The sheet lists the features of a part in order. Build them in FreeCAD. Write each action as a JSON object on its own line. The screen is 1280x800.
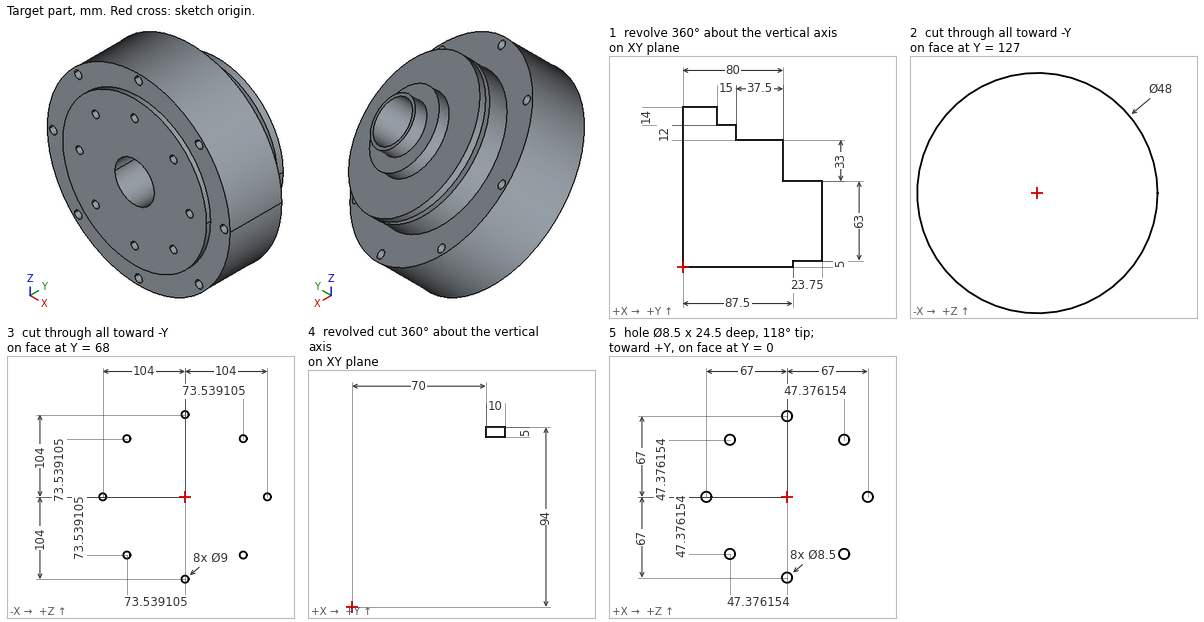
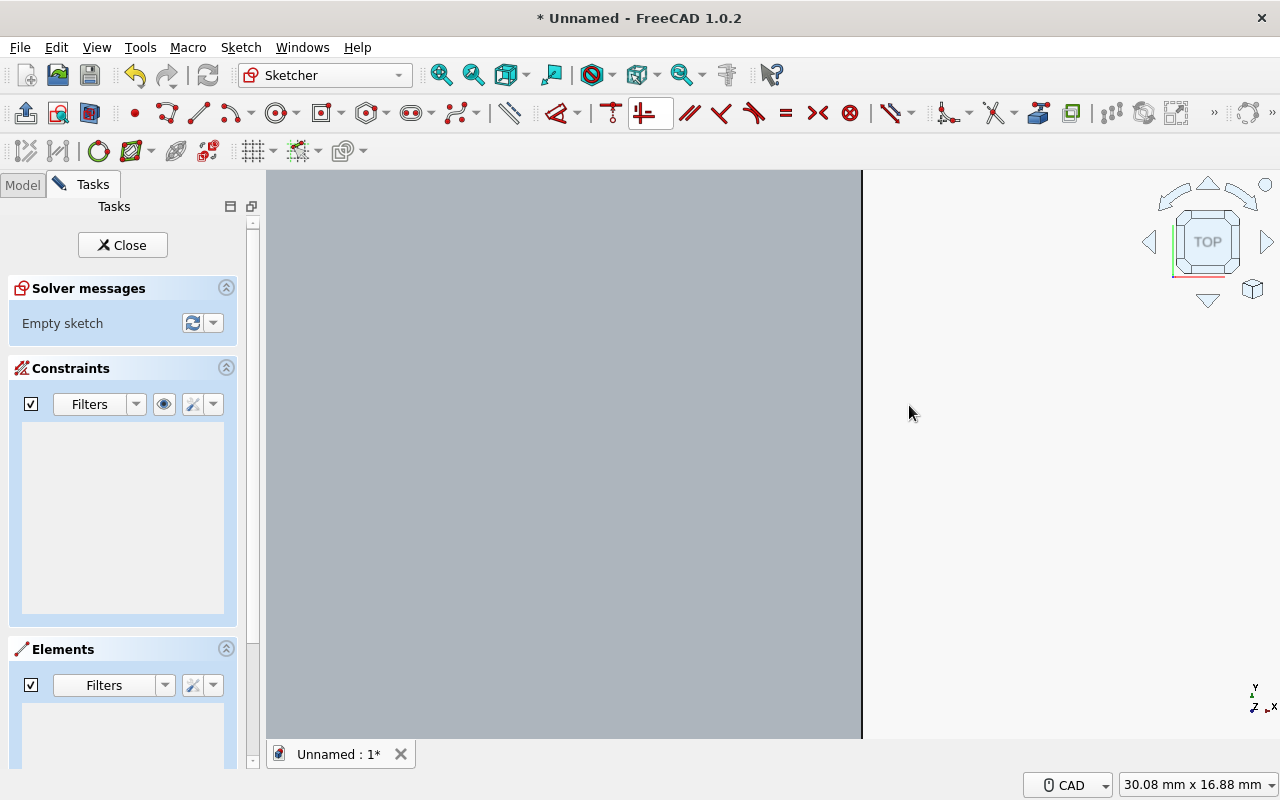
{"action": "scroll", "coordinate": [679, 439], "scroll_direction": "up", "scroll_amount": 3}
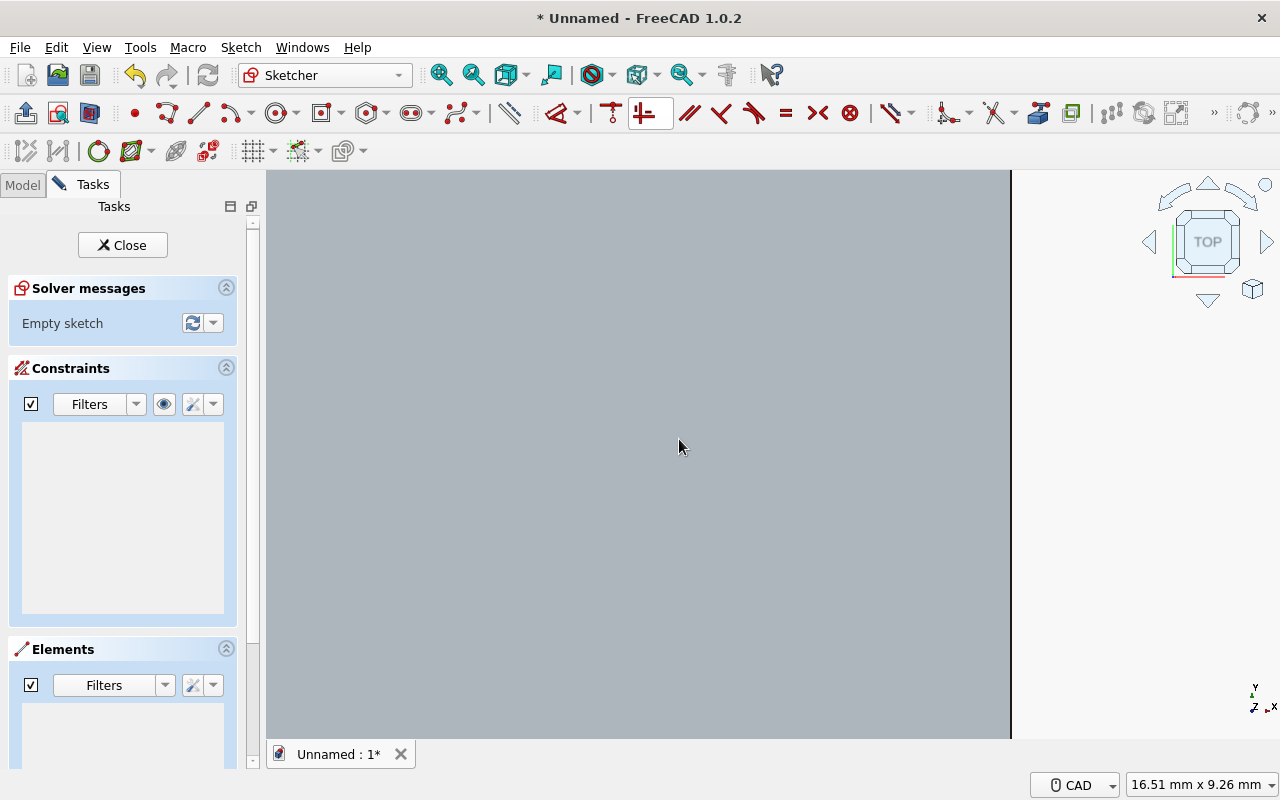
{"action": "left_click", "coordinate": [344, 114]}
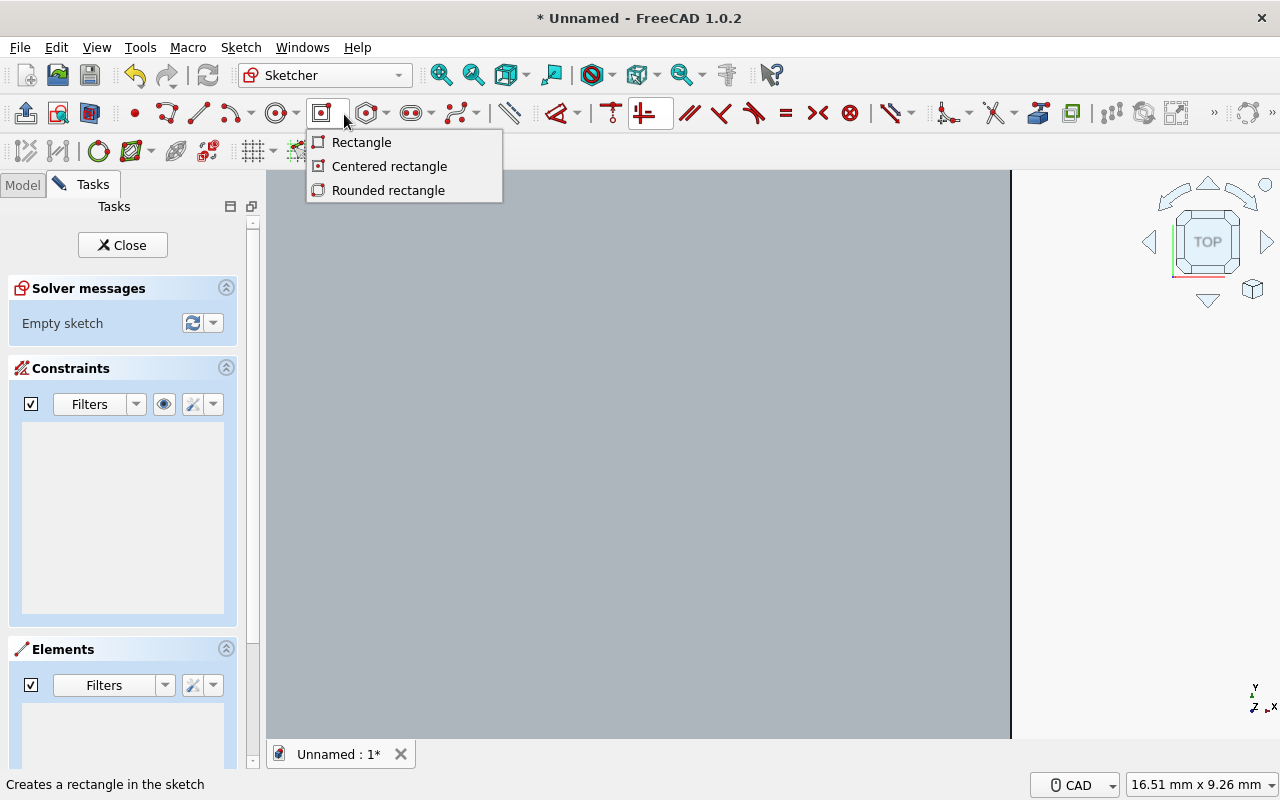
{"action": "left_click", "coordinate": [404, 142]}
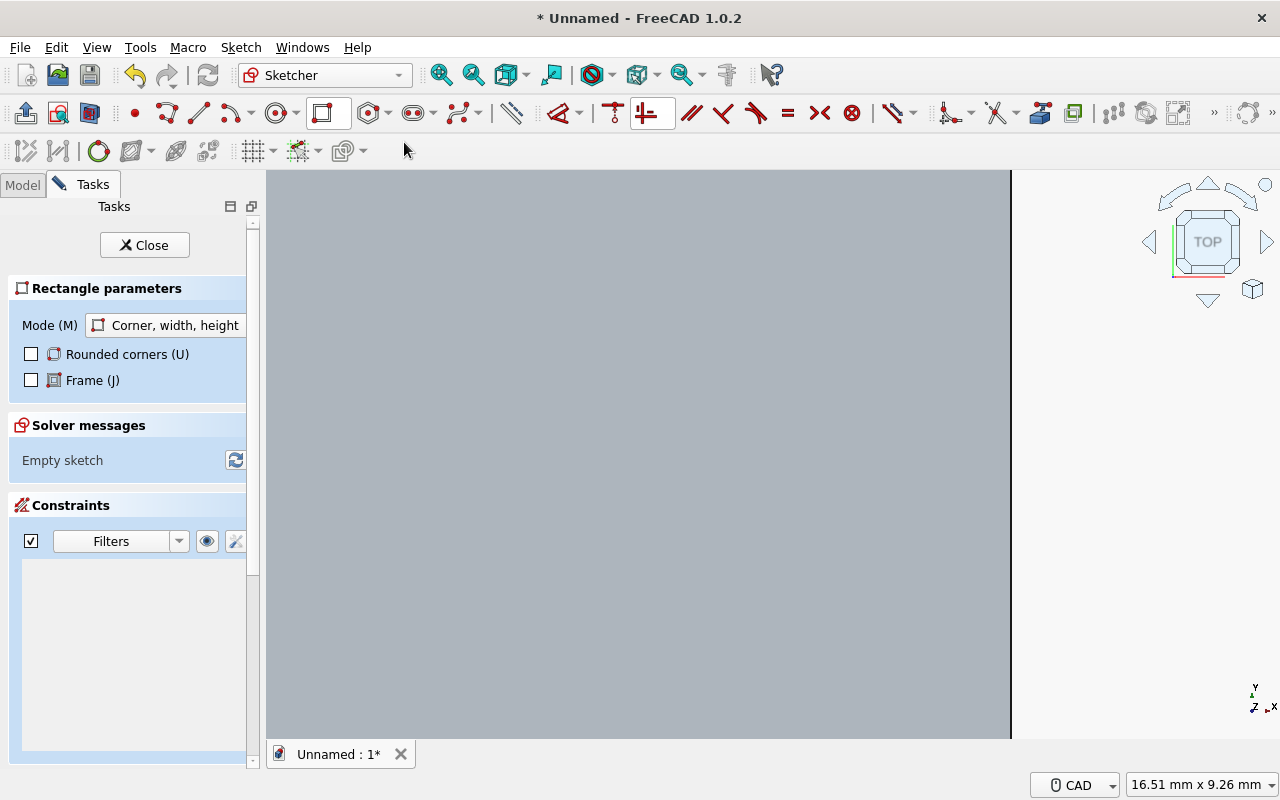
{"action": "left_click", "coordinate": [397, 301]}
{"action": "left_click", "coordinate": [1011, 608]}
{"action": "key", "text": "Escape"}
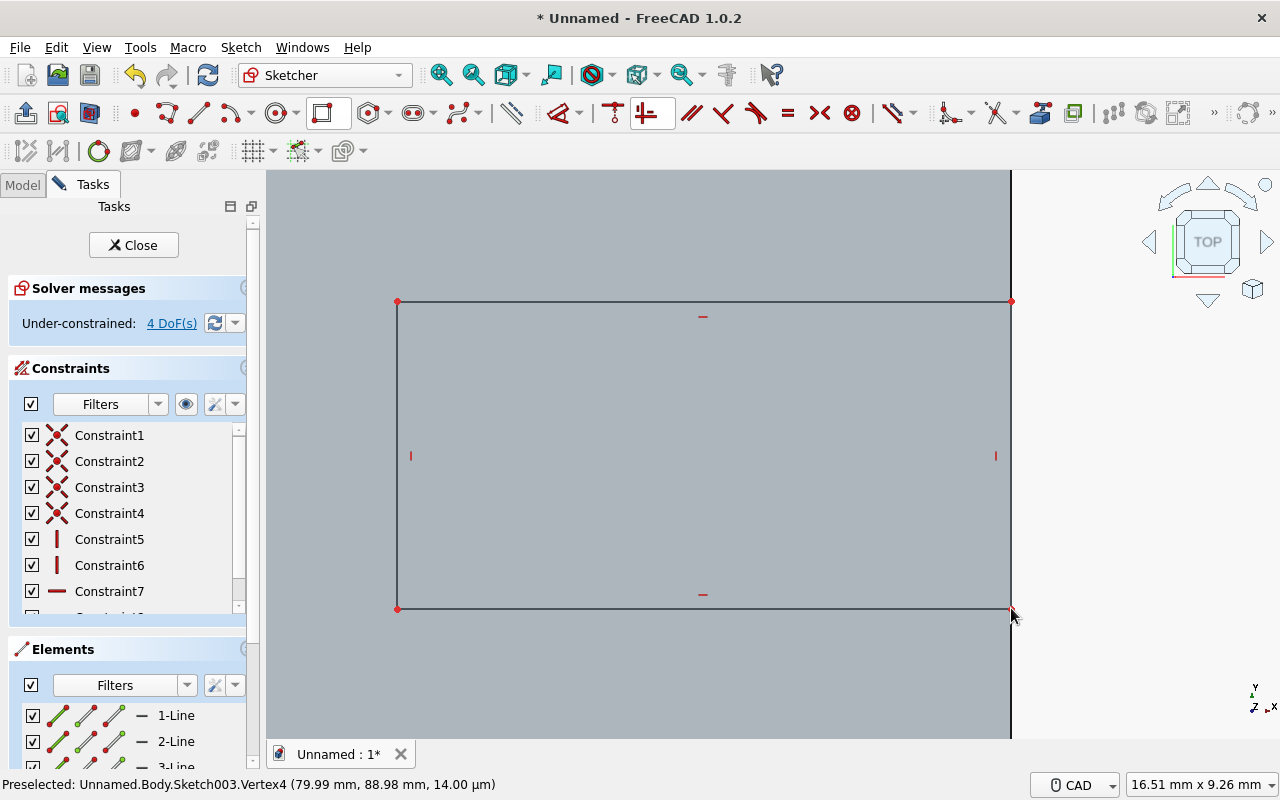
{"action": "left_click", "coordinate": [558, 114]}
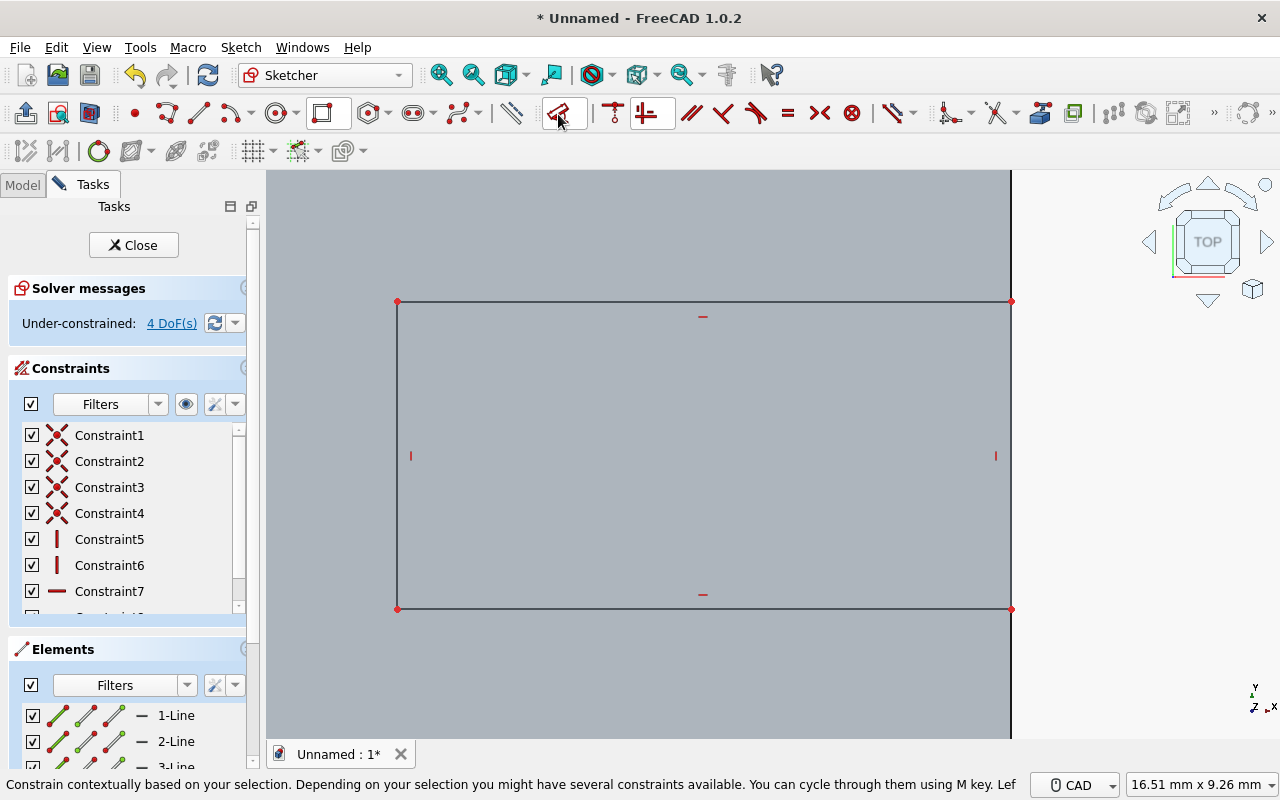
{"action": "left_click", "coordinate": [397, 394]}
{"action": "left_click", "coordinate": [363, 456]}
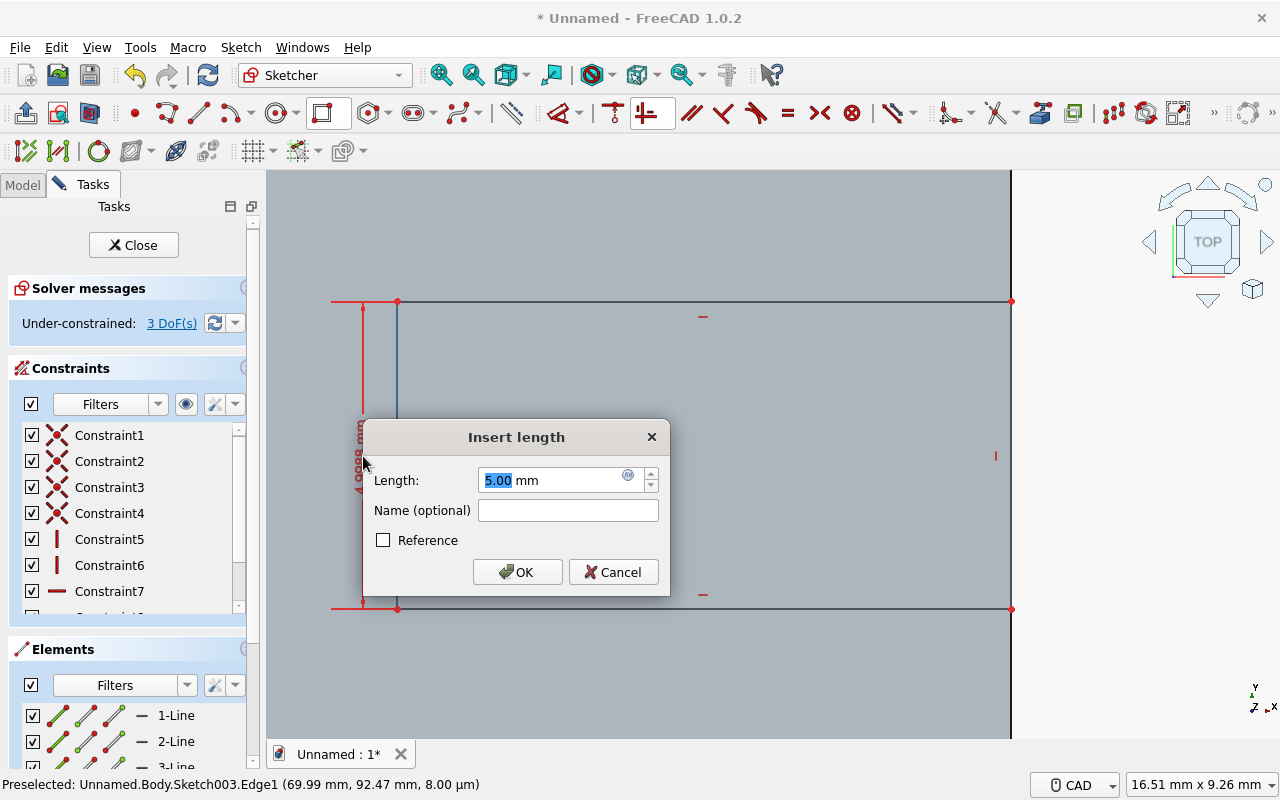
{"action": "type", "text": "5"}
{"action": "key", "text": "Return"}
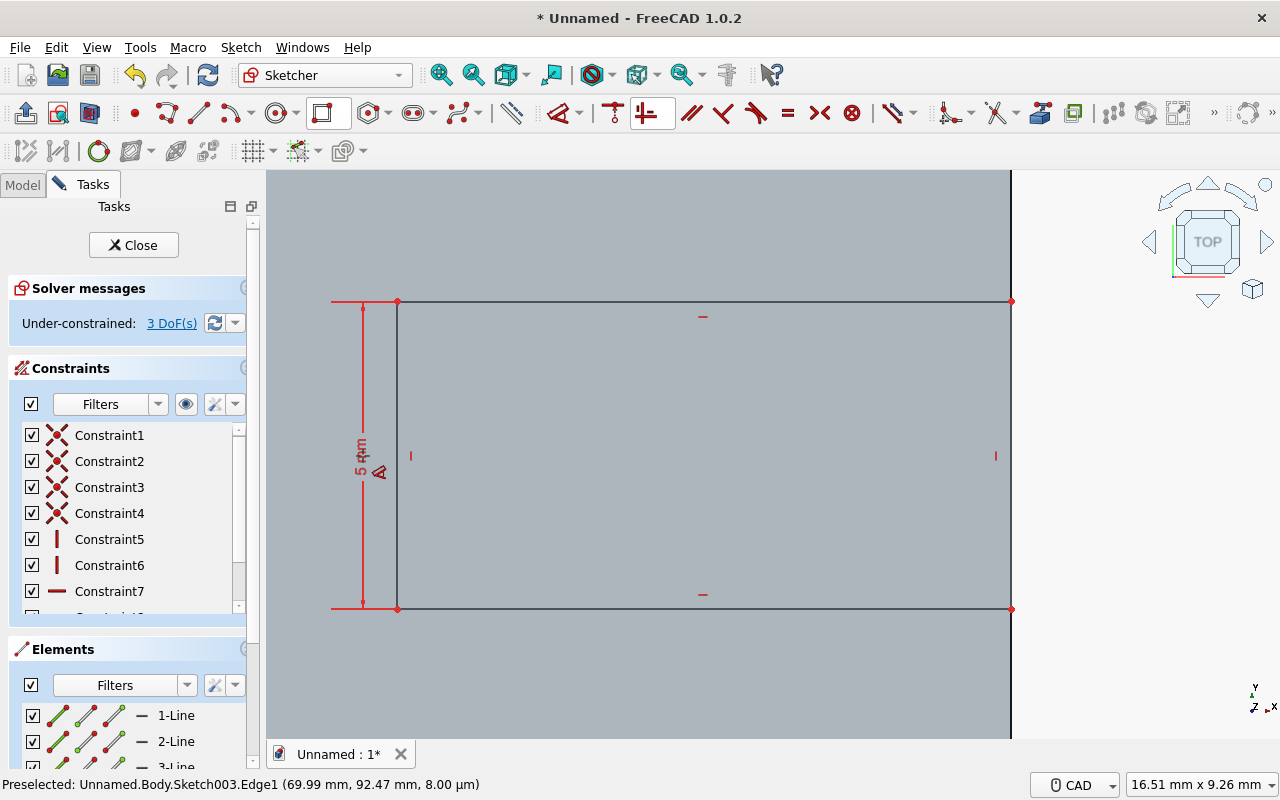
{"action": "left_click", "coordinate": [581, 609]}
{"action": "left_click", "coordinate": [704, 643]}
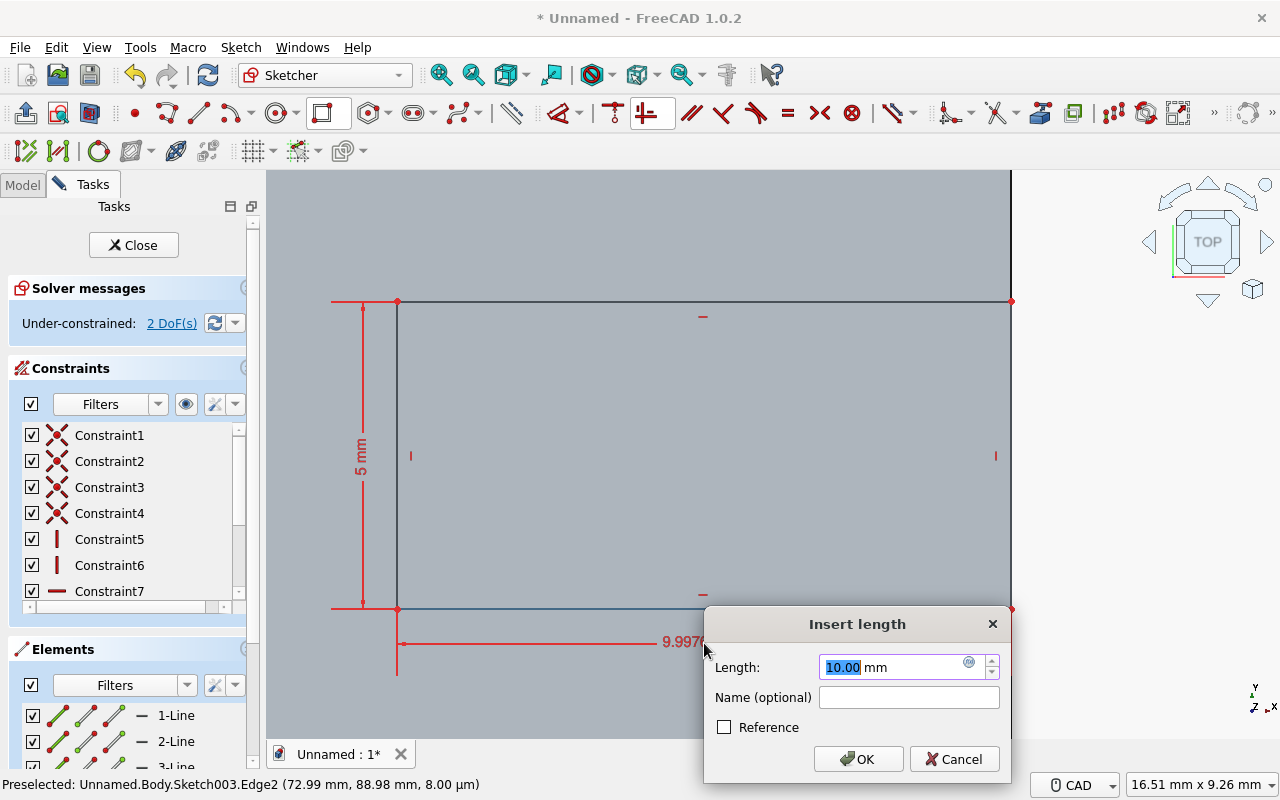
{"action": "type", "text": "10"}
{"action": "key", "text": "Return"}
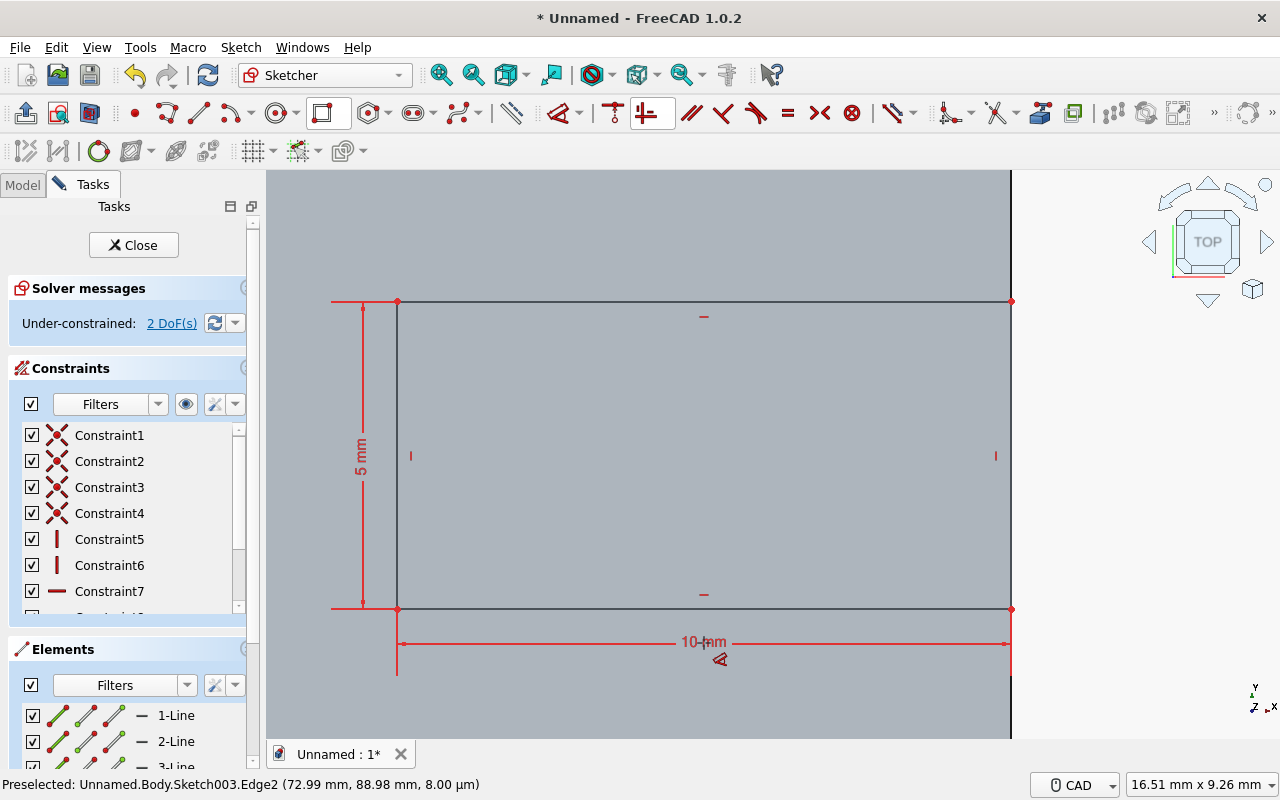
{"action": "left_click", "coordinate": [397, 302]}
{"action": "left_click", "coordinate": [346, 268]}